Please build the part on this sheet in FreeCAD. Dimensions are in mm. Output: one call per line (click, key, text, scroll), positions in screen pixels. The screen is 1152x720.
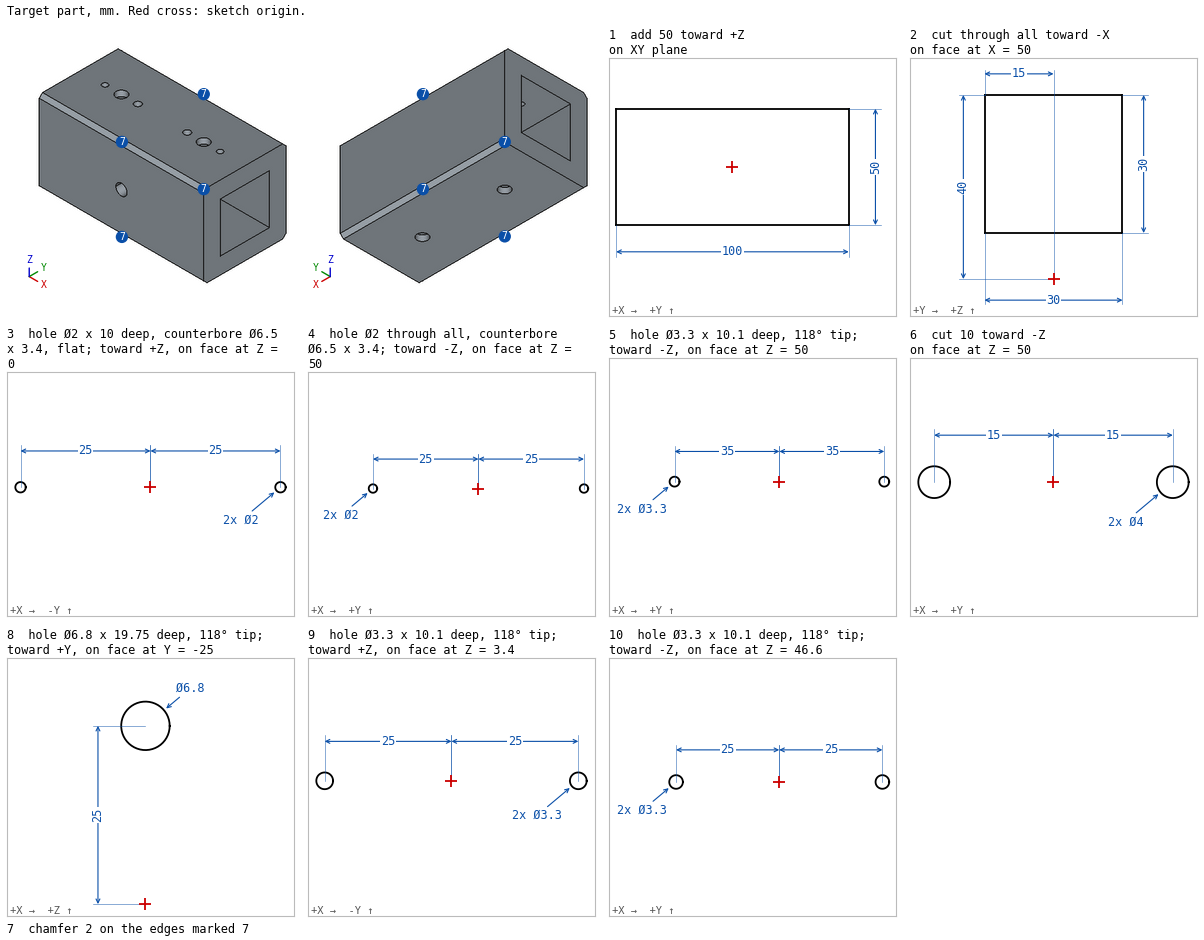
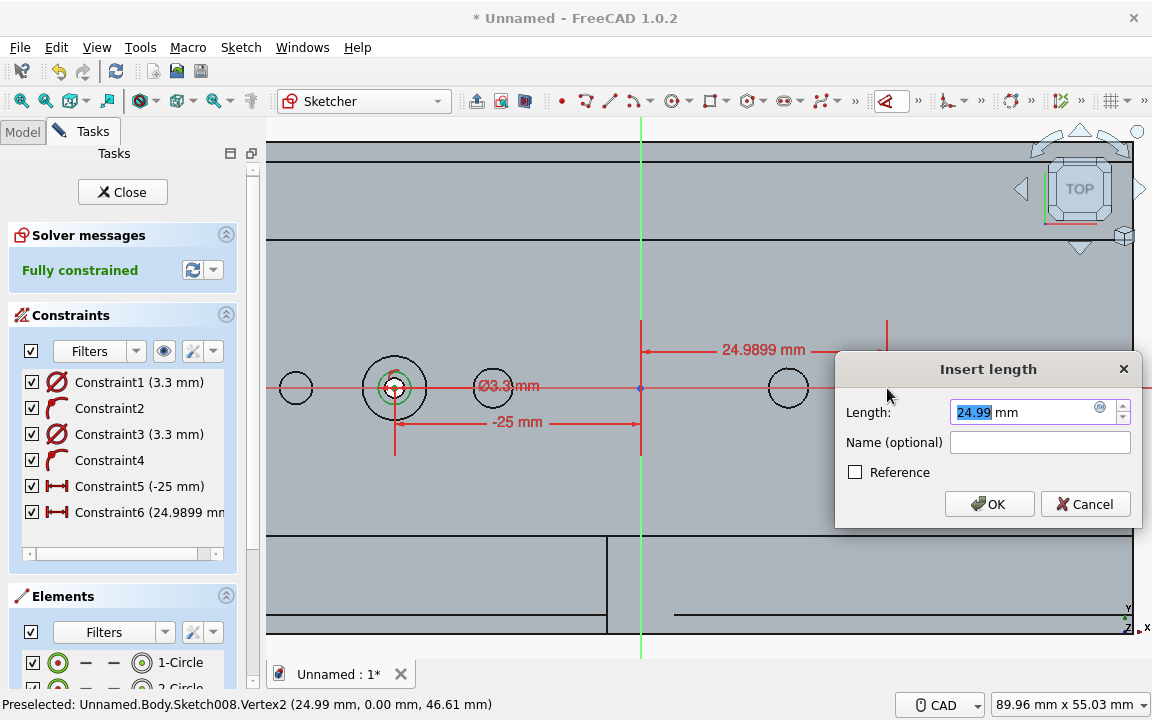
text(25)
key(Return)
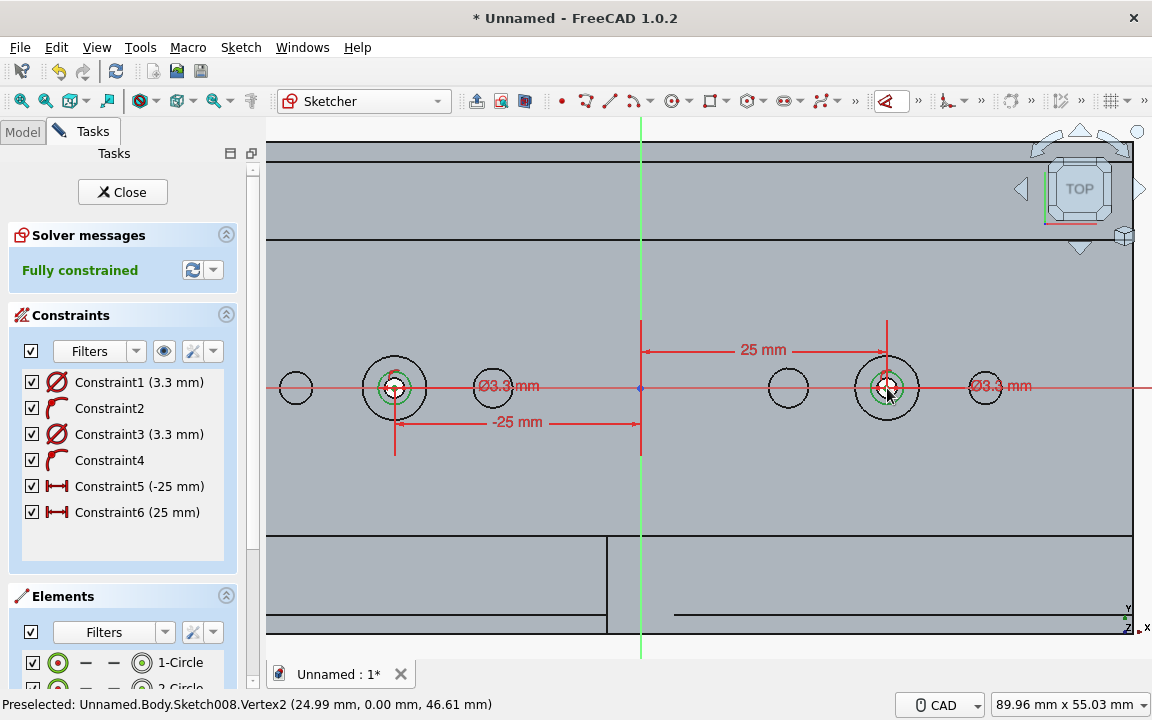
click(123, 192)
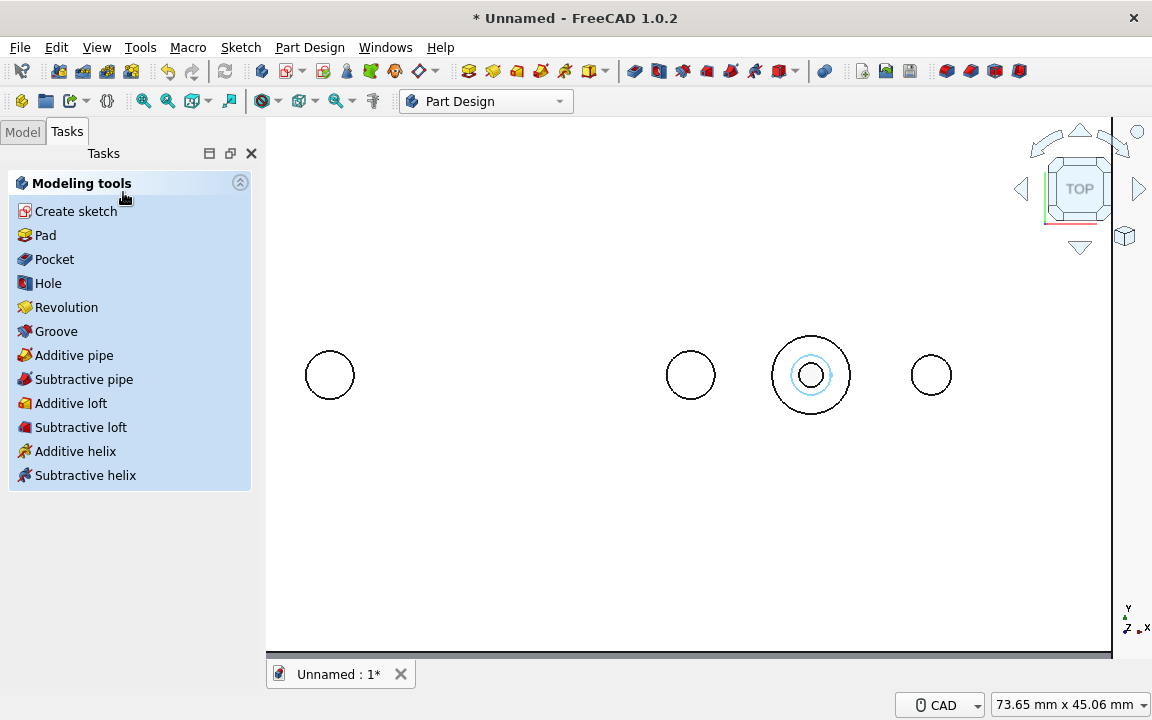
click(660, 72)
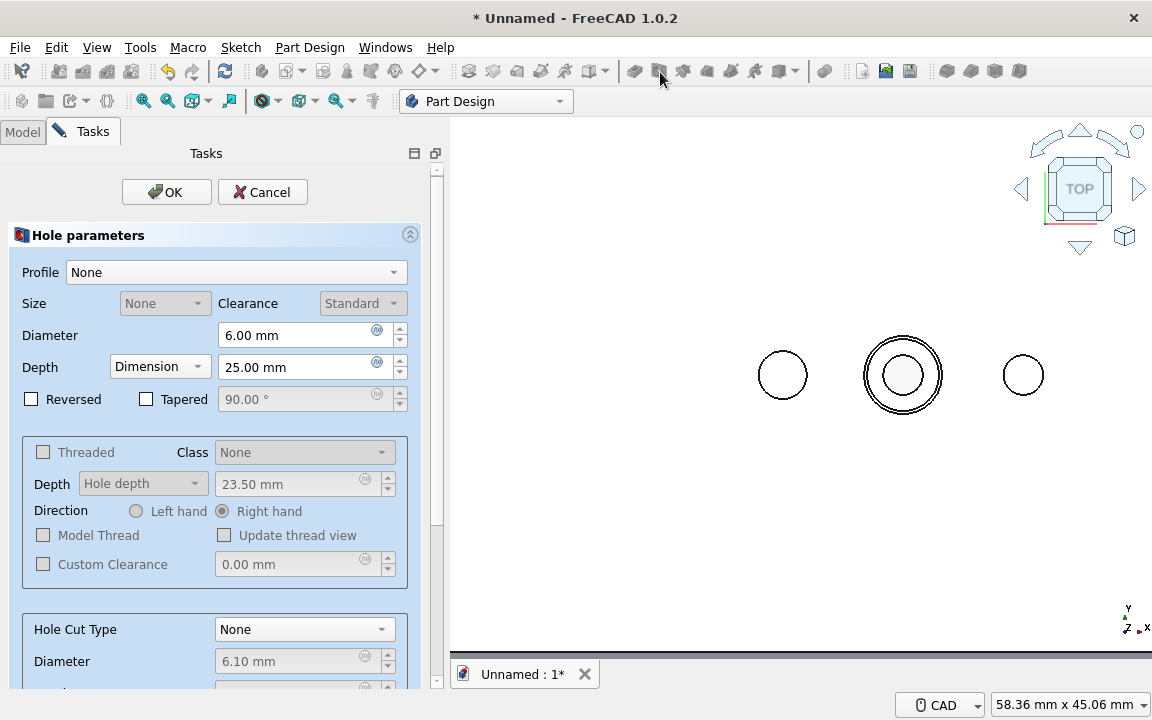
triple_click(305, 335)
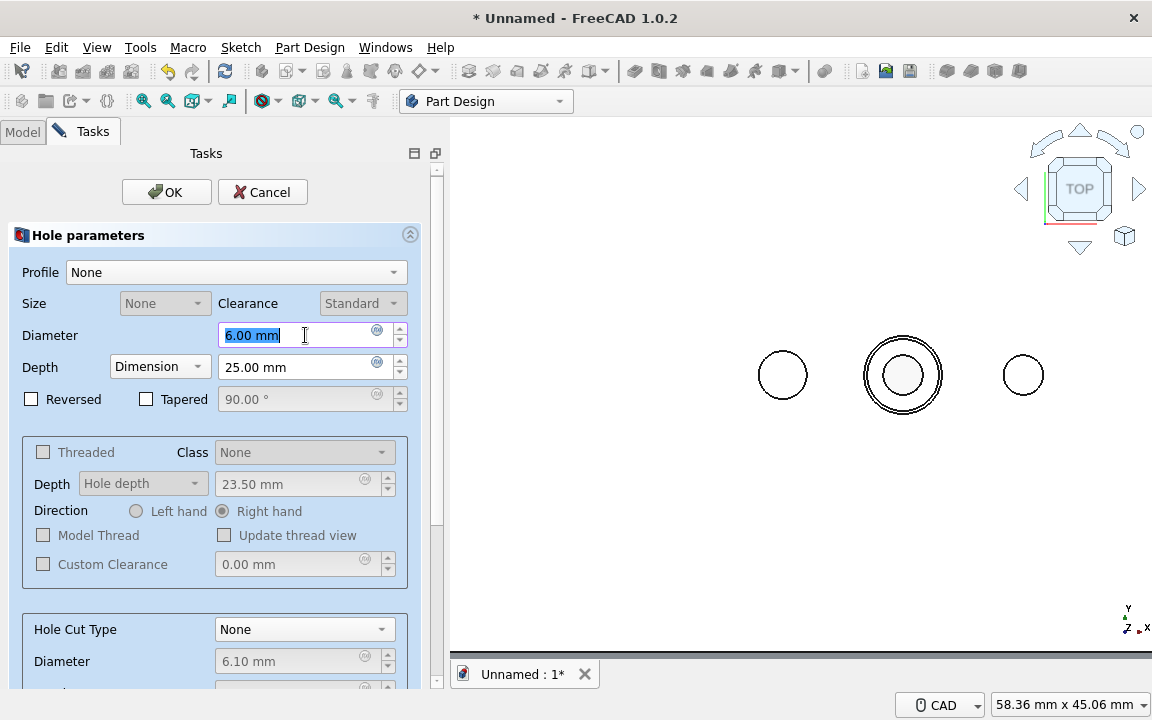
text(3.3)
key(Tab)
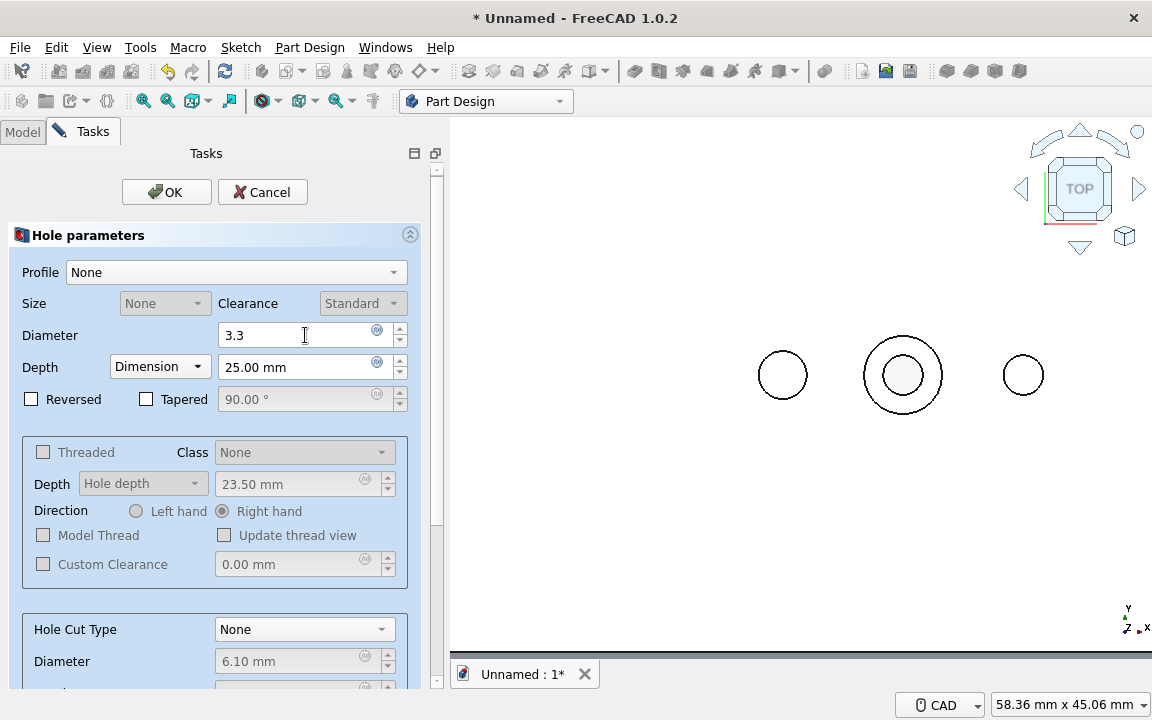
triple_click(305, 367)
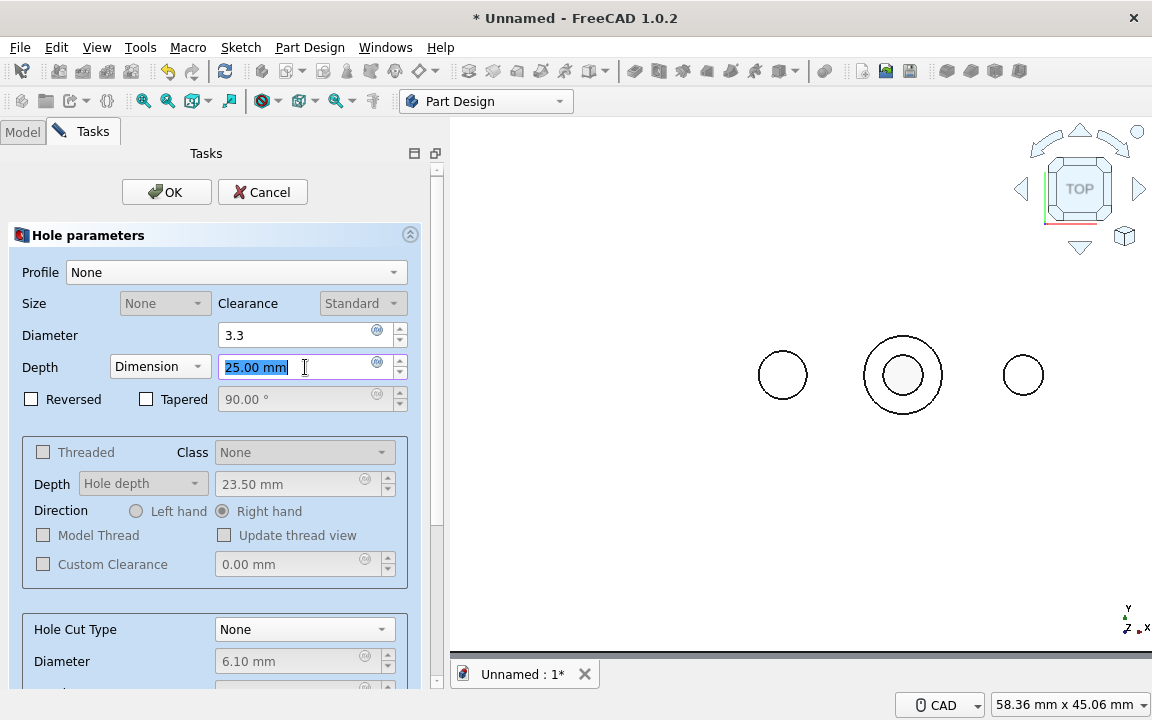
text(10.1)
key(Tab)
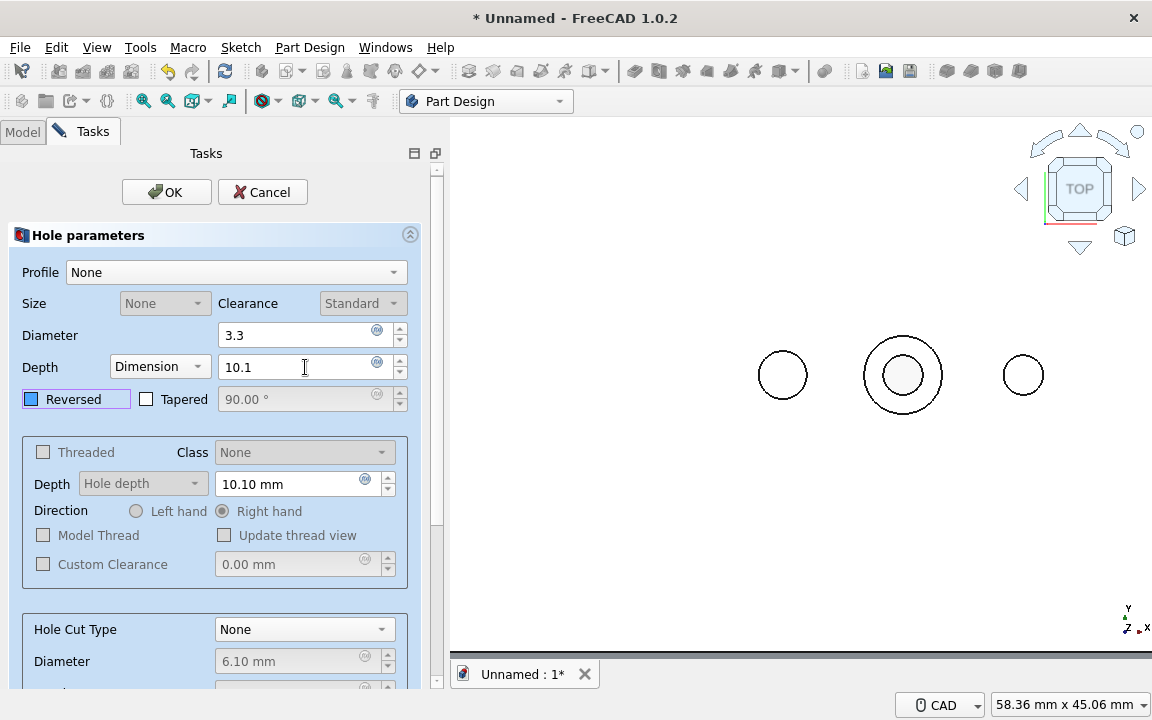
click(167, 192)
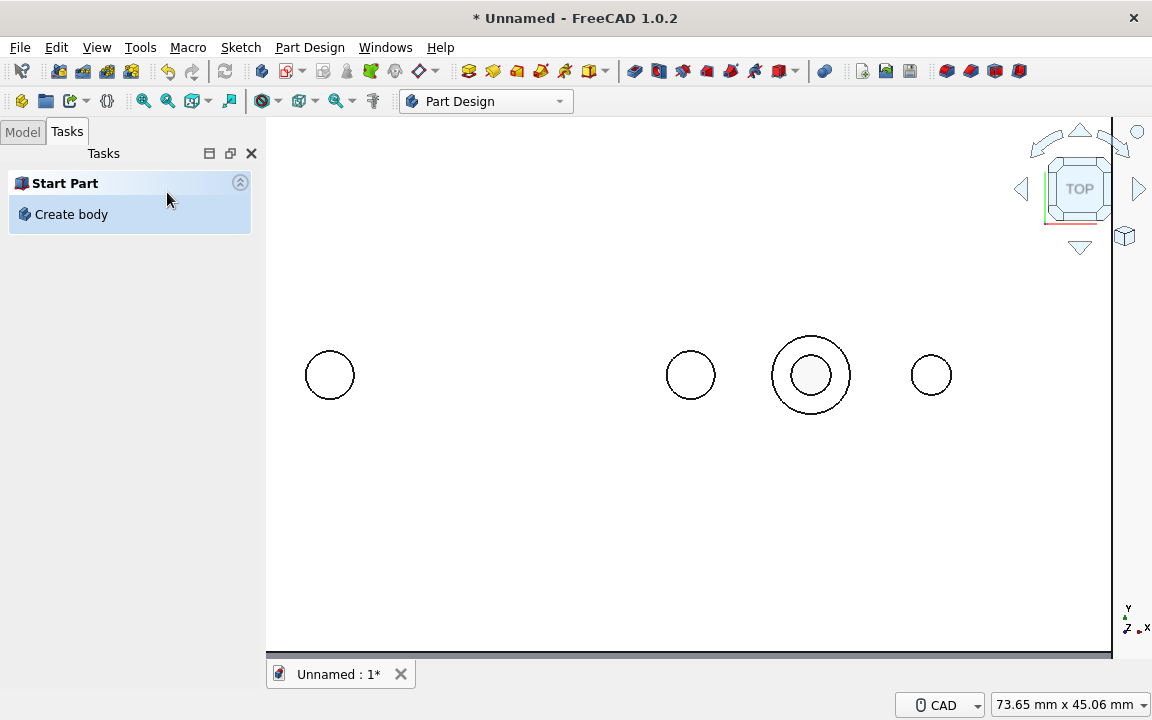
key(0)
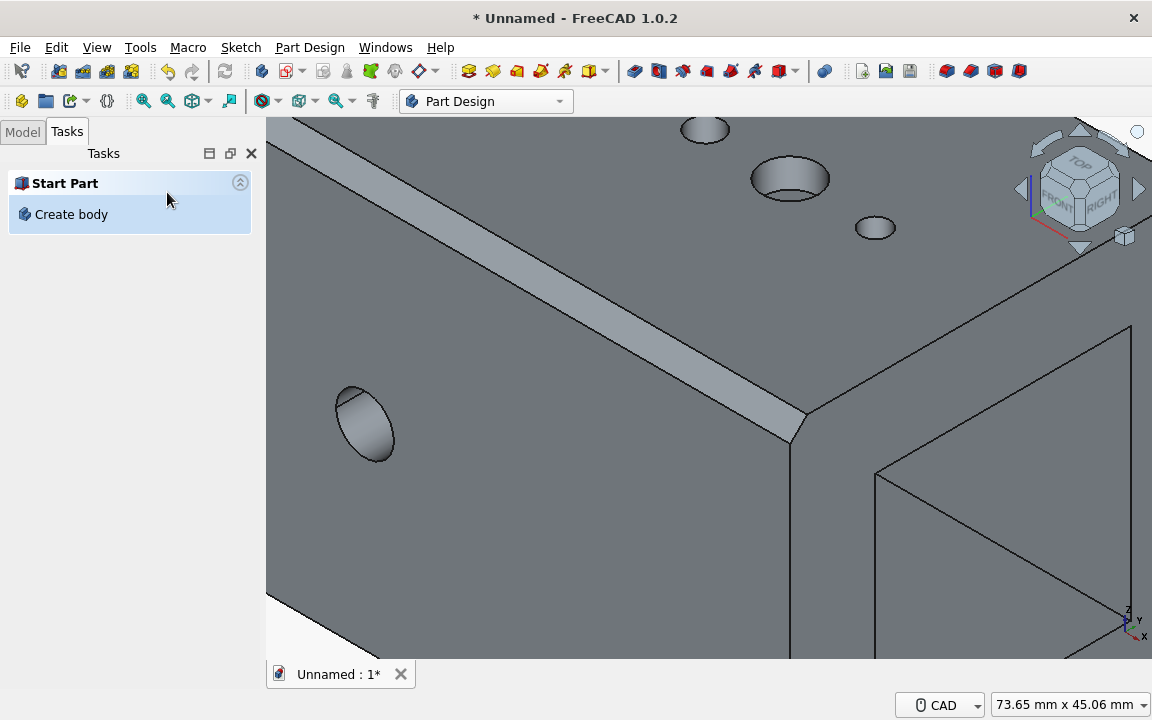
click(144, 102)